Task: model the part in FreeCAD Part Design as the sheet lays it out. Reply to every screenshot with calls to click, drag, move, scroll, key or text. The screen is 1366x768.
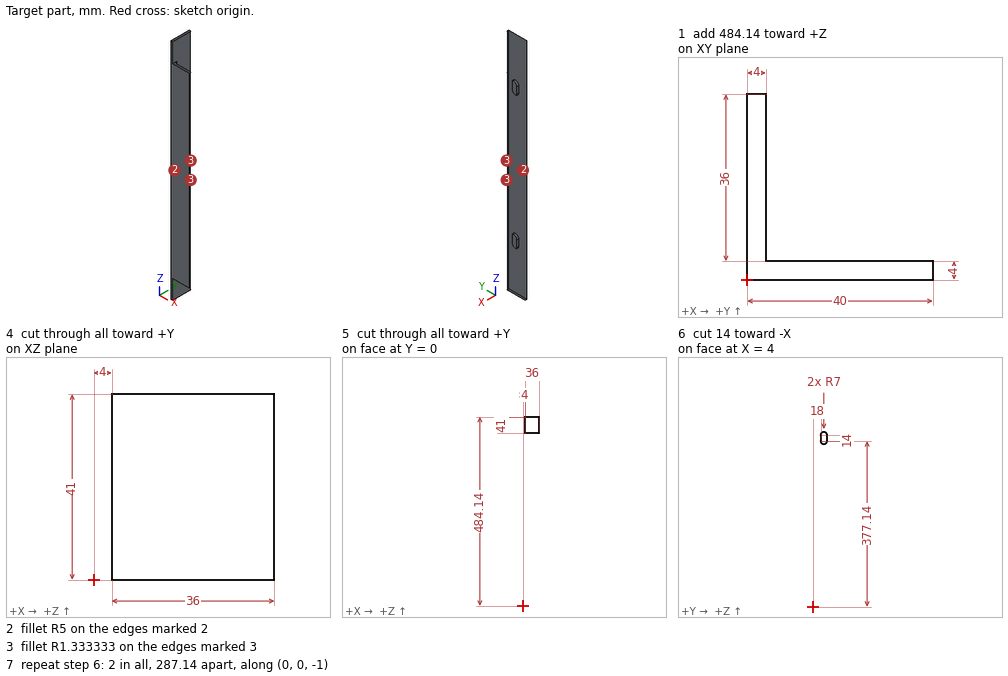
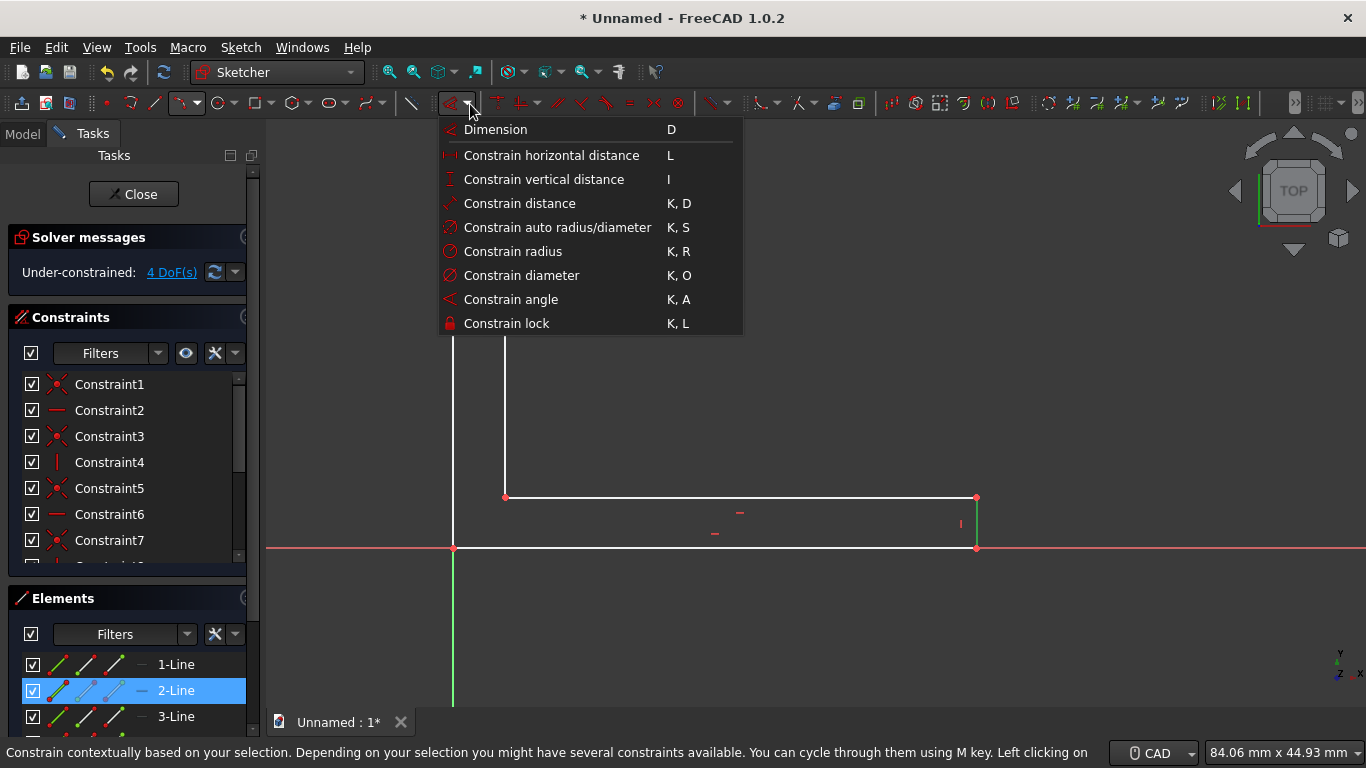
click(591, 179)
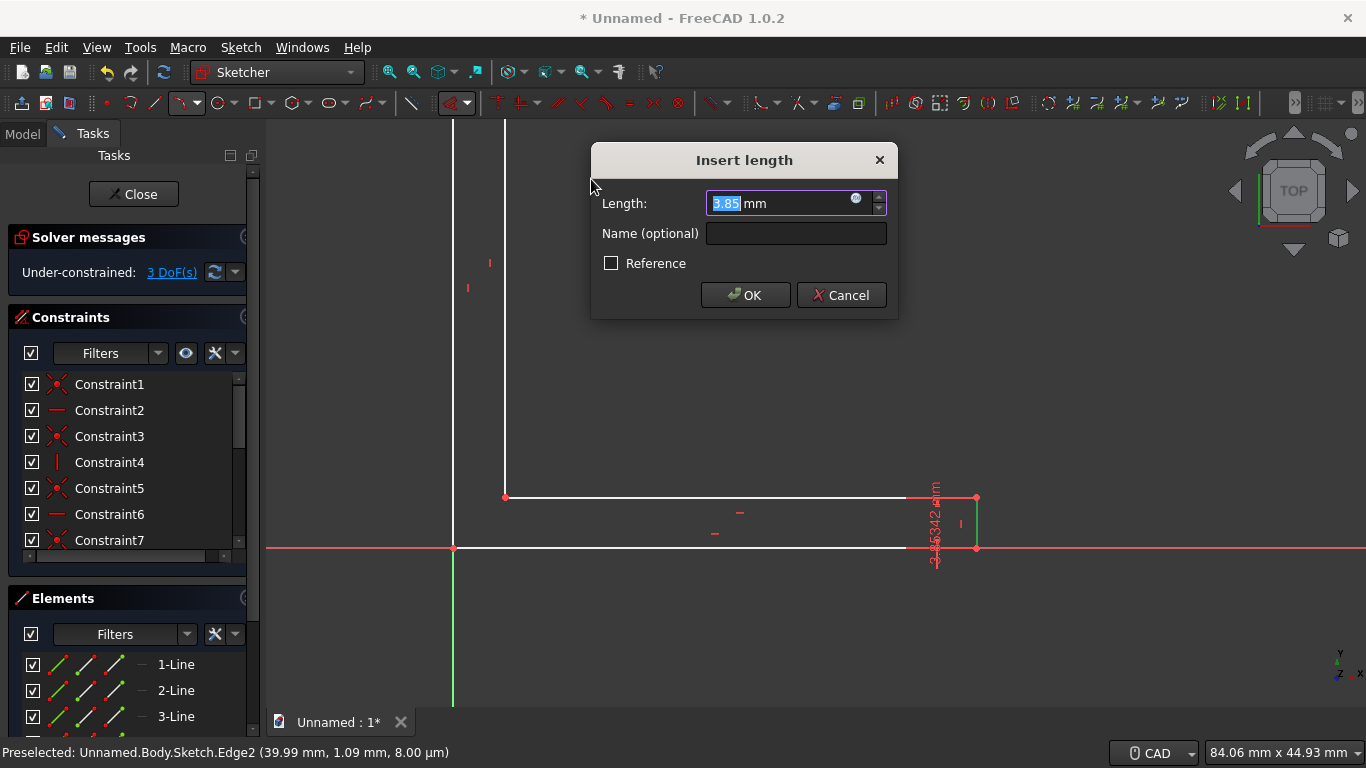
text(4)
key(Return)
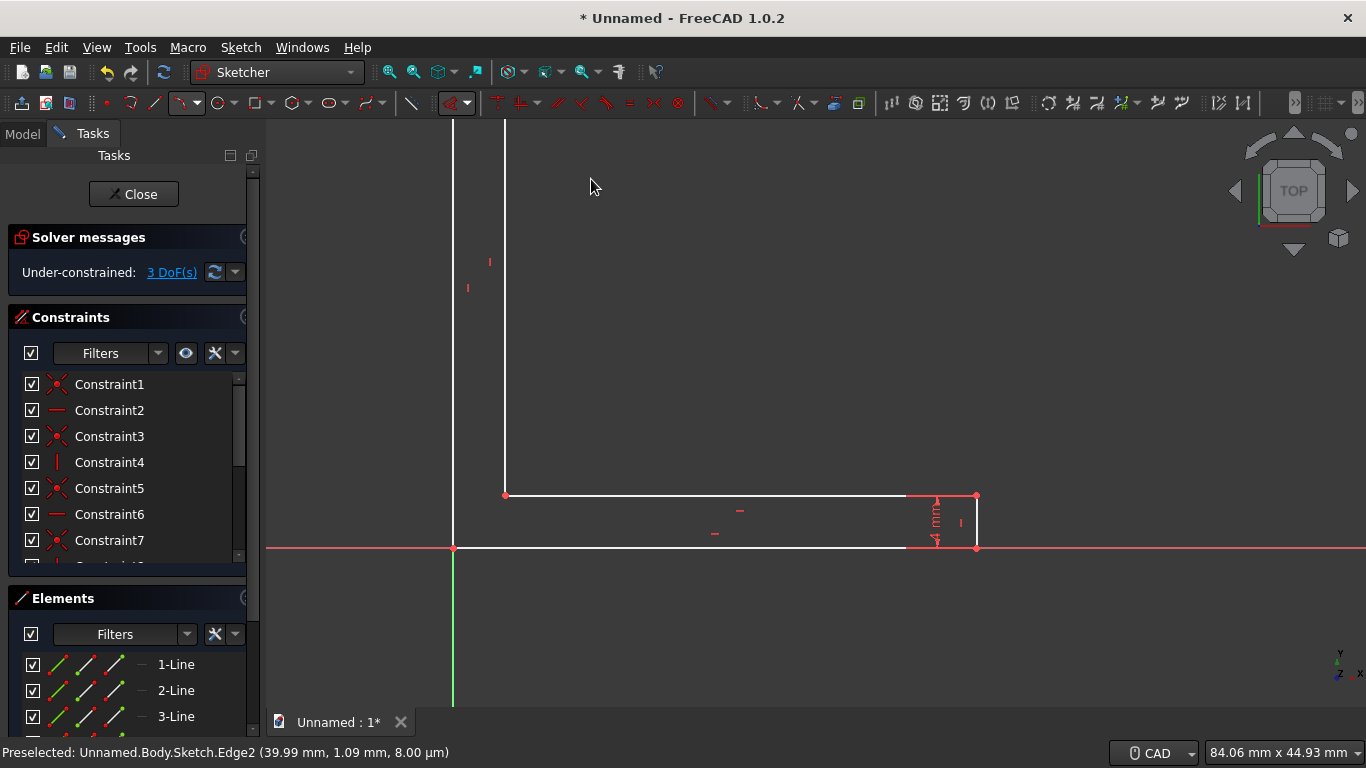
scroll(813, 670, down, 2)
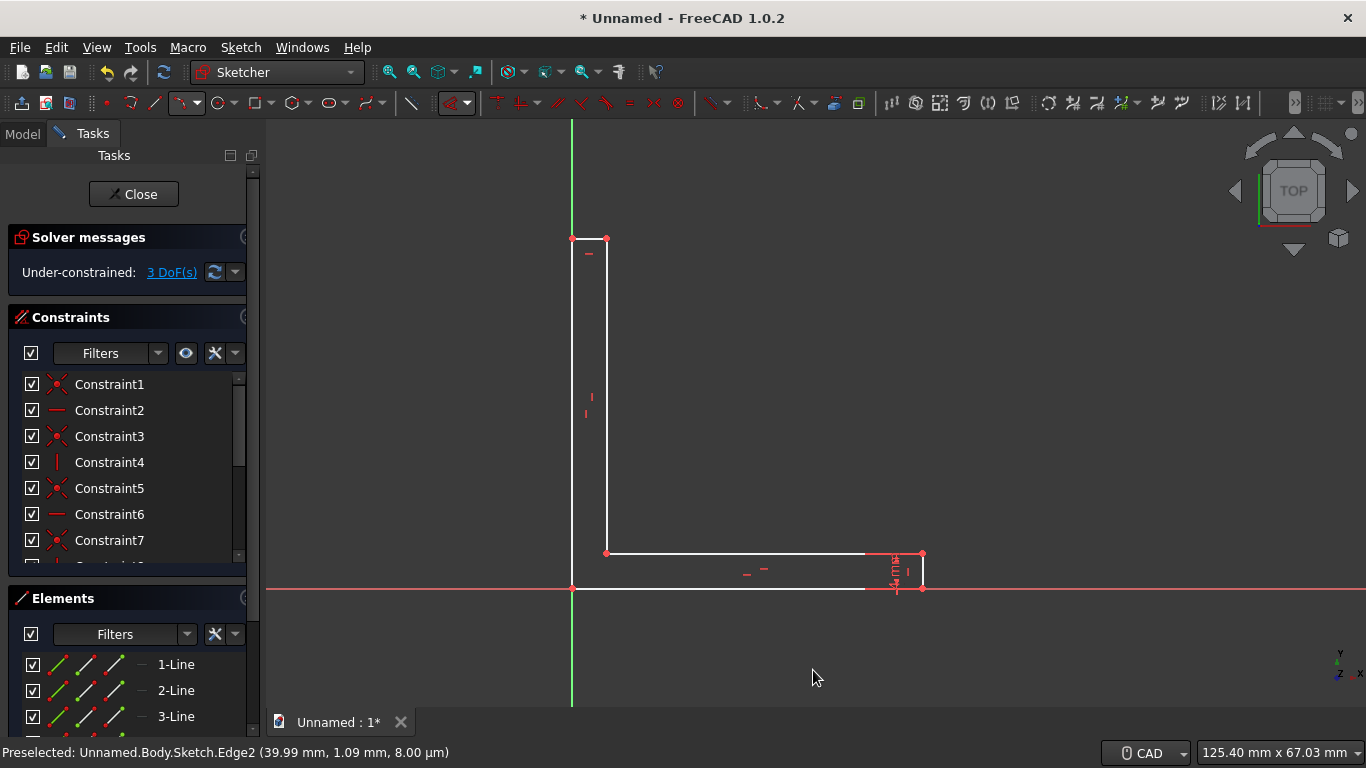
scroll(596, 239, up, 2)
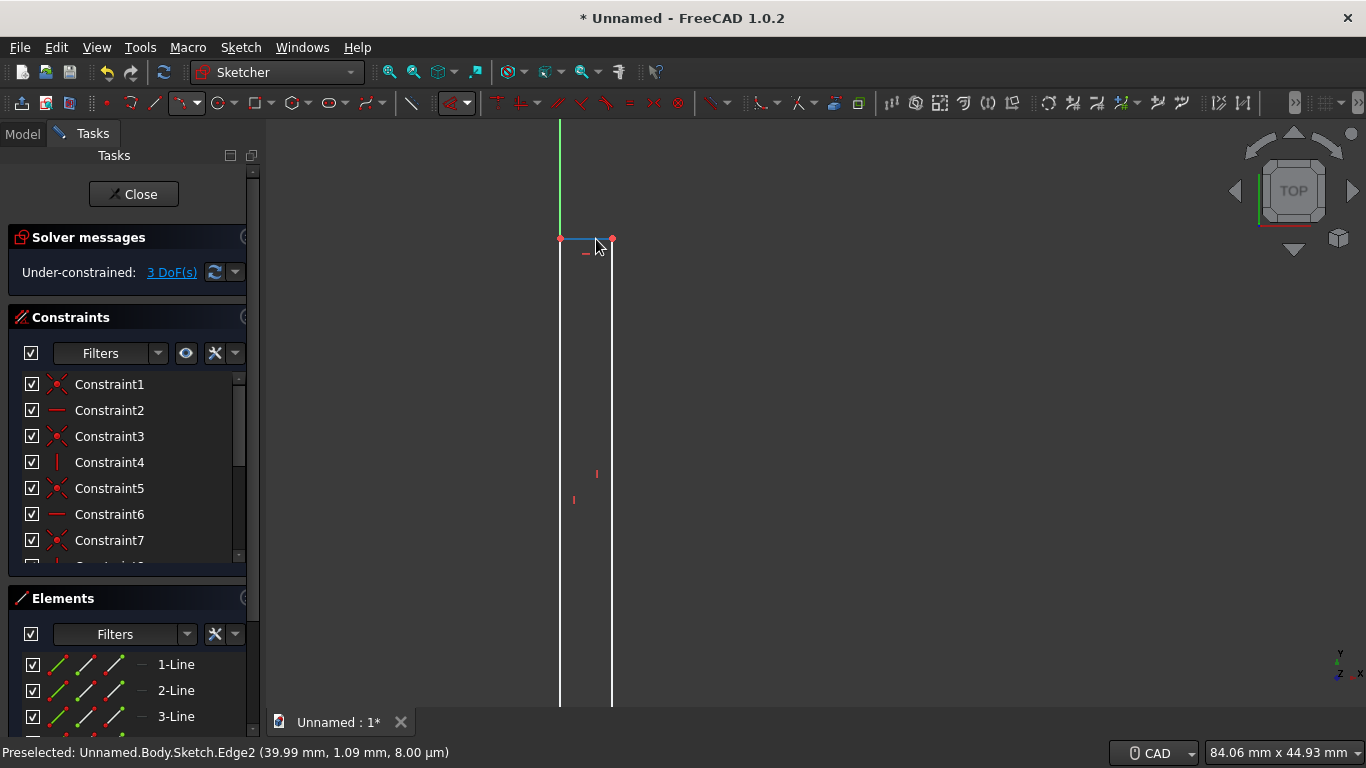
click(597, 239)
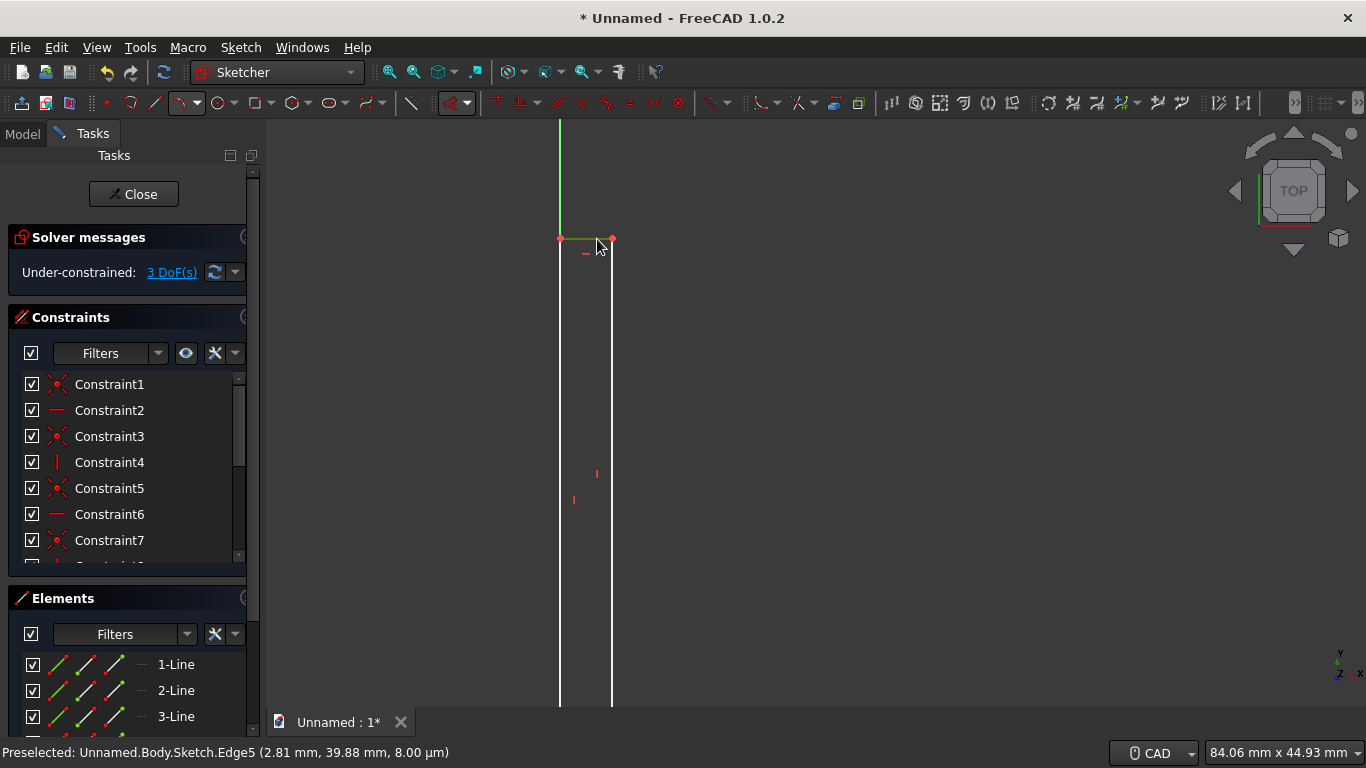
key(l)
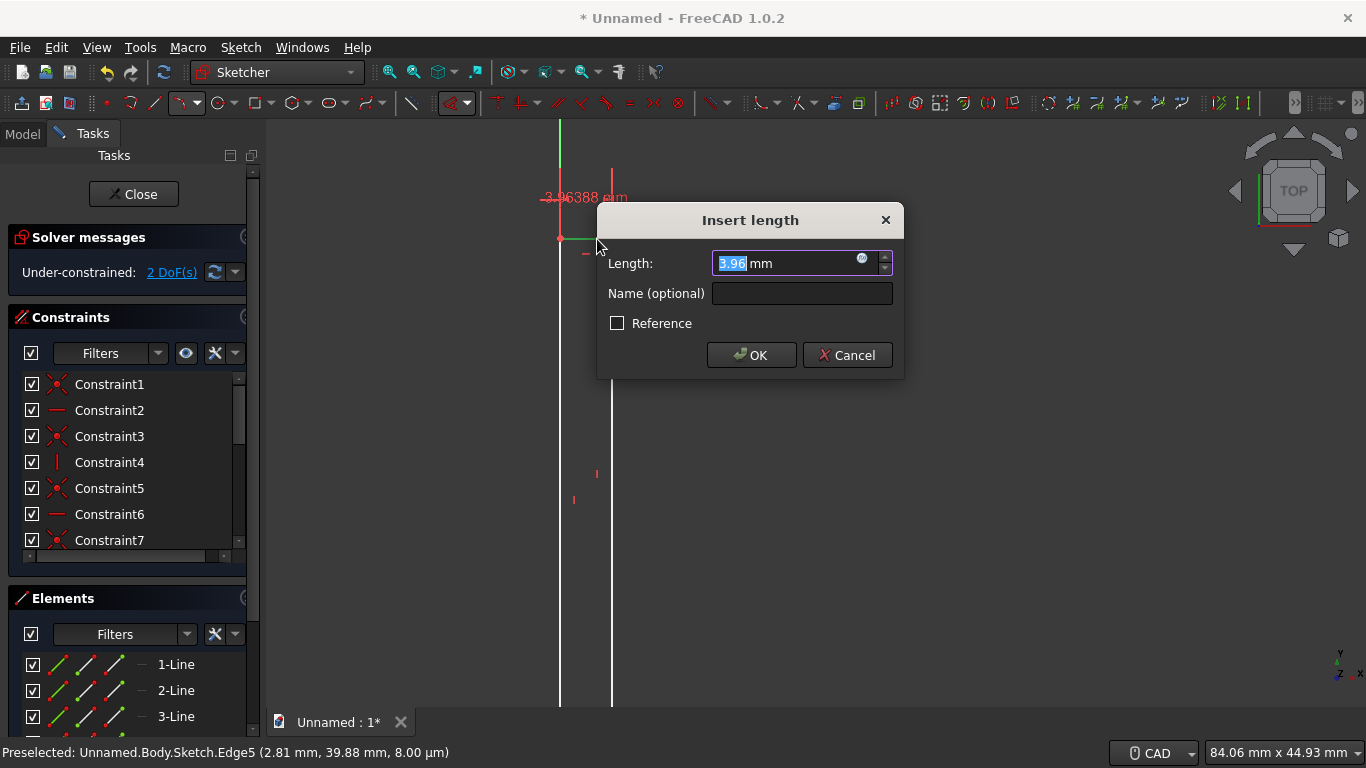
text(4)
key(Return)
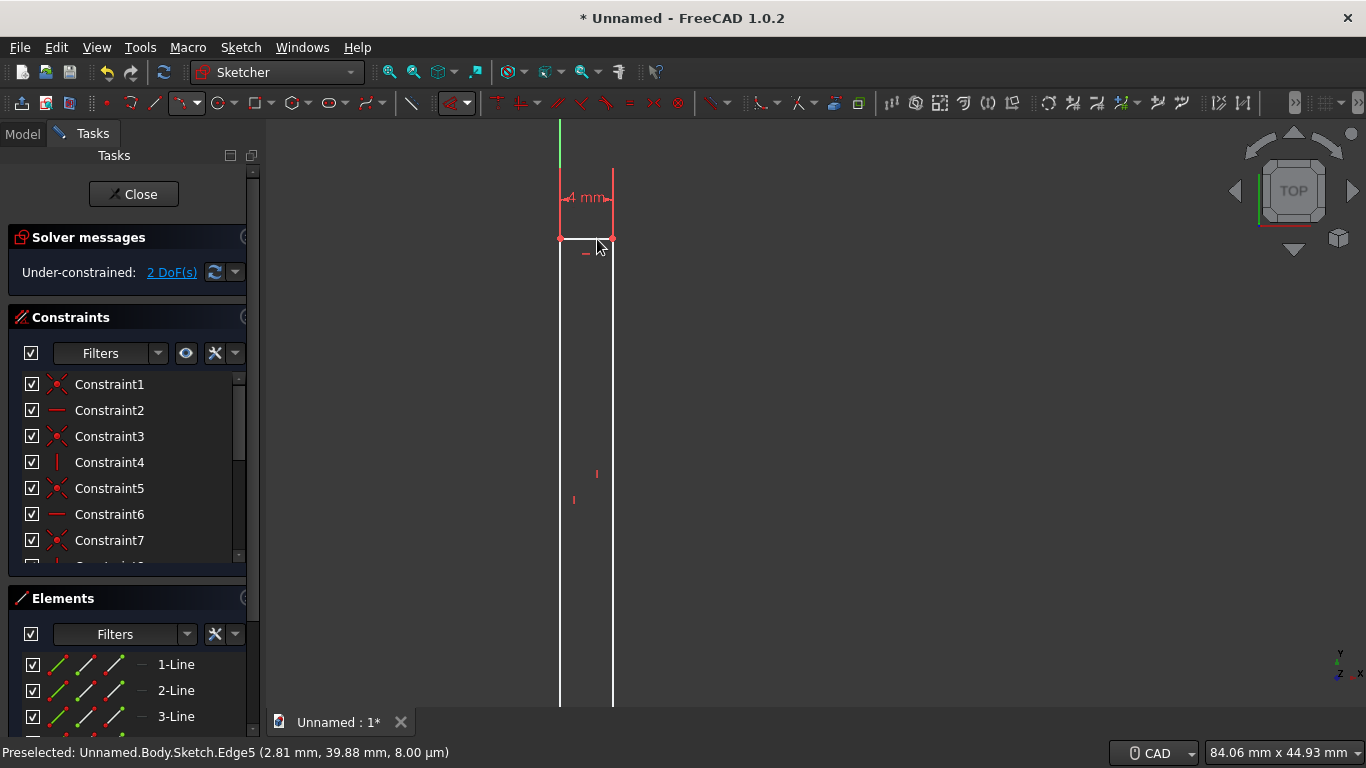
scroll(596, 238, down, 2)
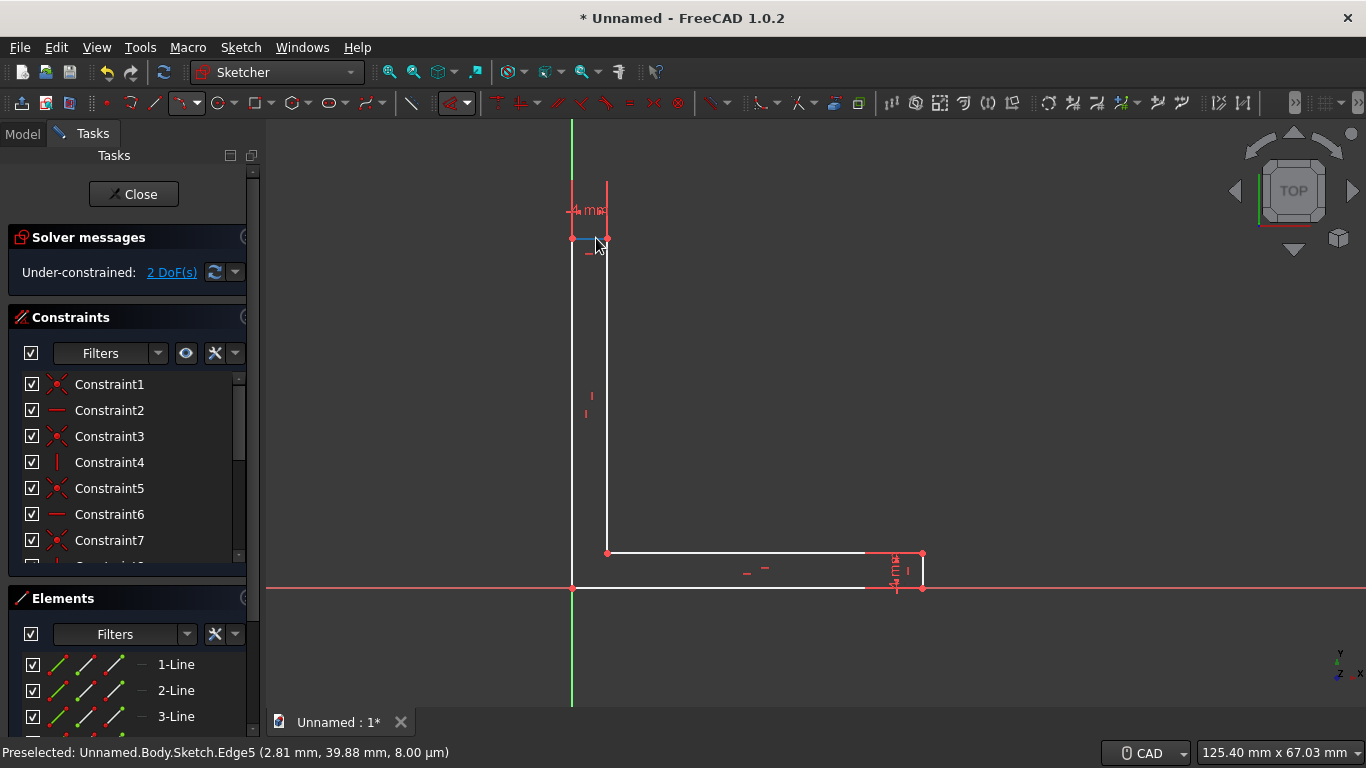
click(677, 588)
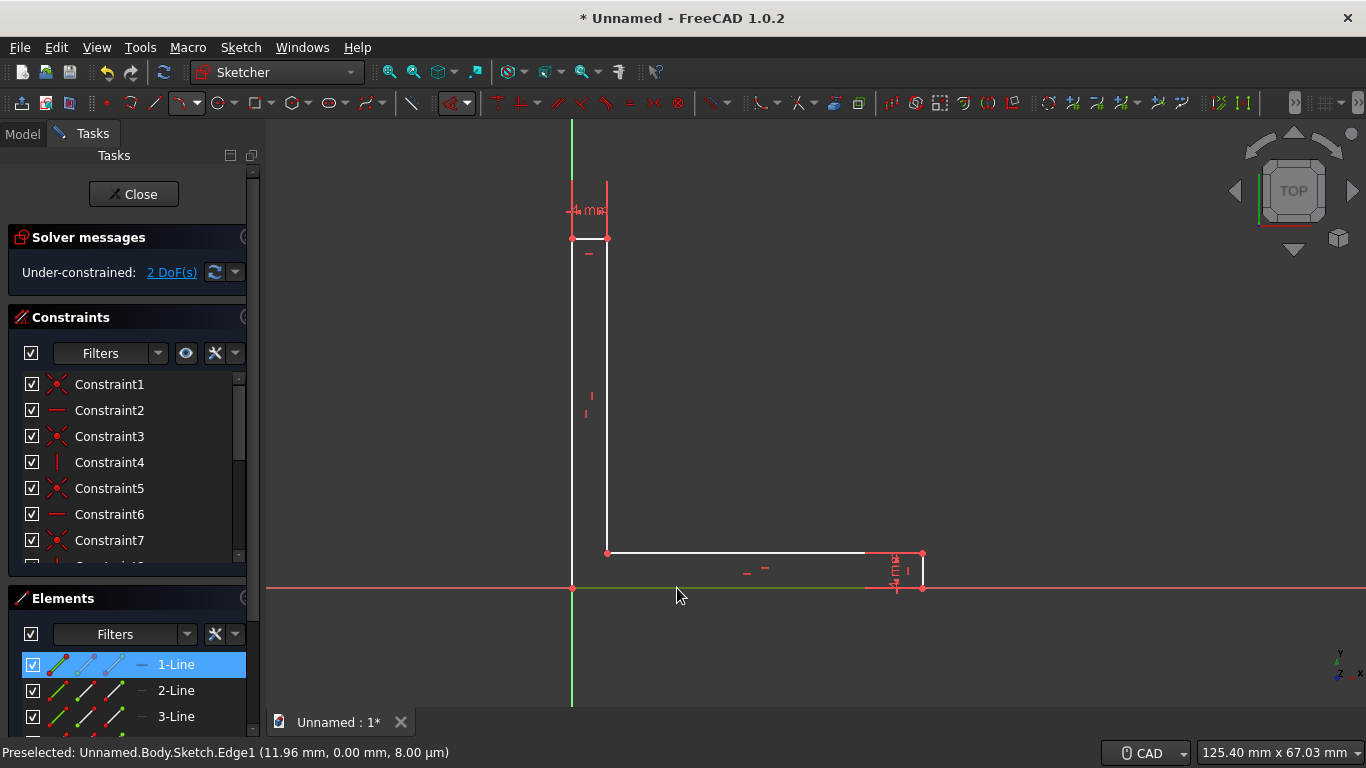
click(470, 104)